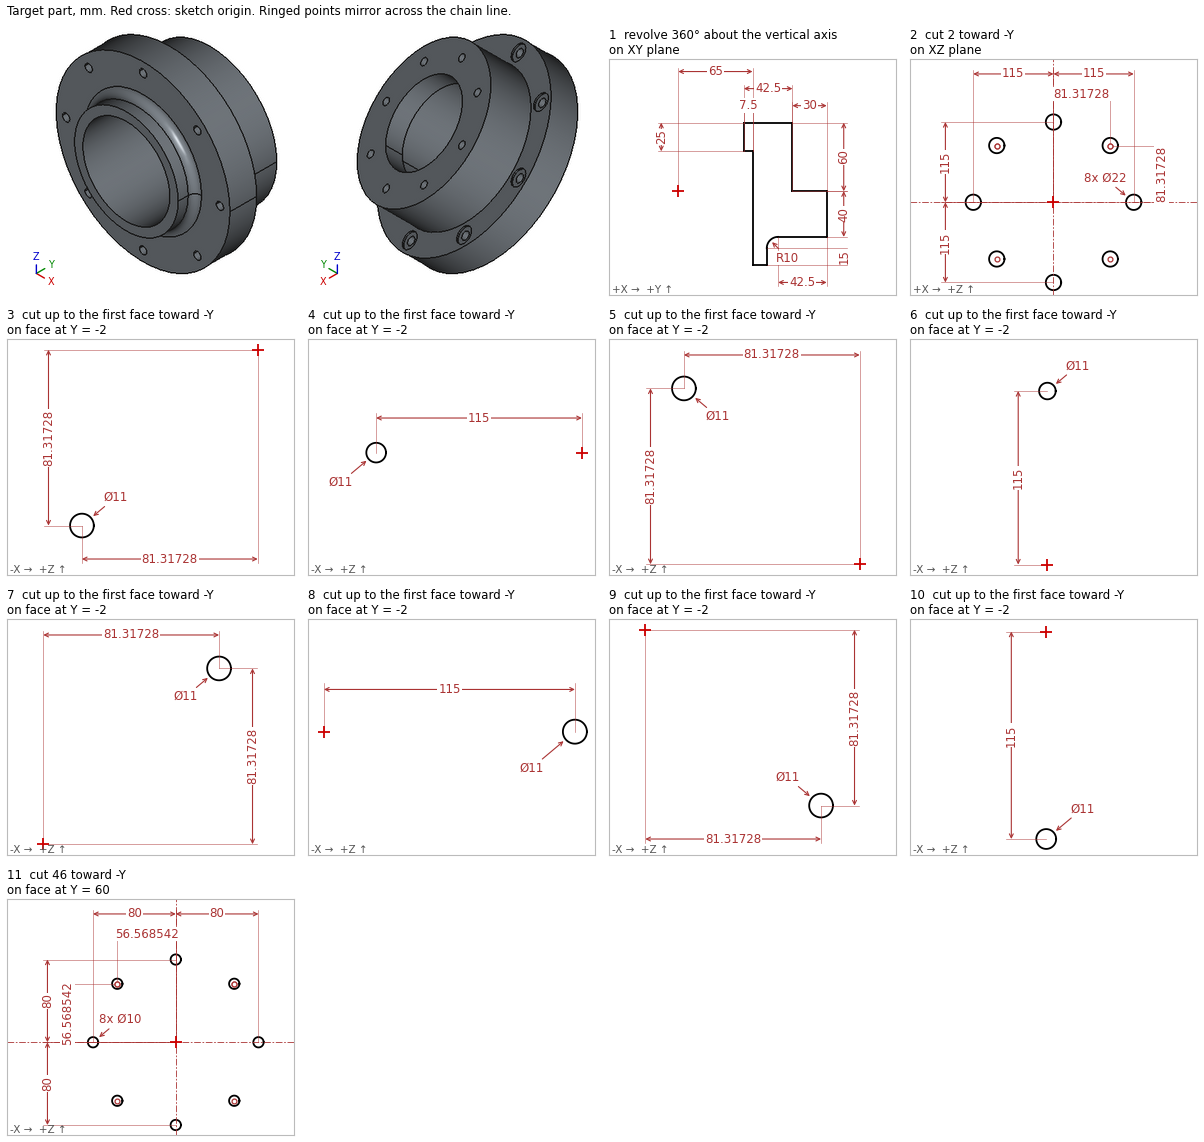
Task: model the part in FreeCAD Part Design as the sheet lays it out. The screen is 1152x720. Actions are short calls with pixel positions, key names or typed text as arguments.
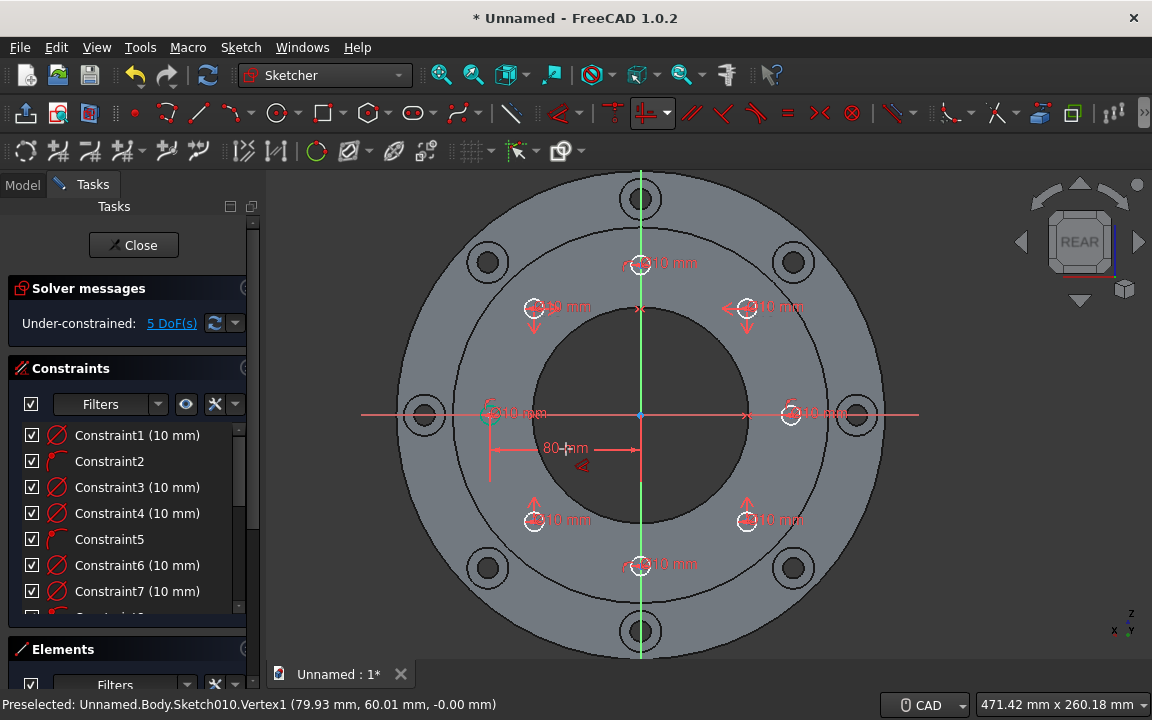
click(641, 265)
click(675, 340)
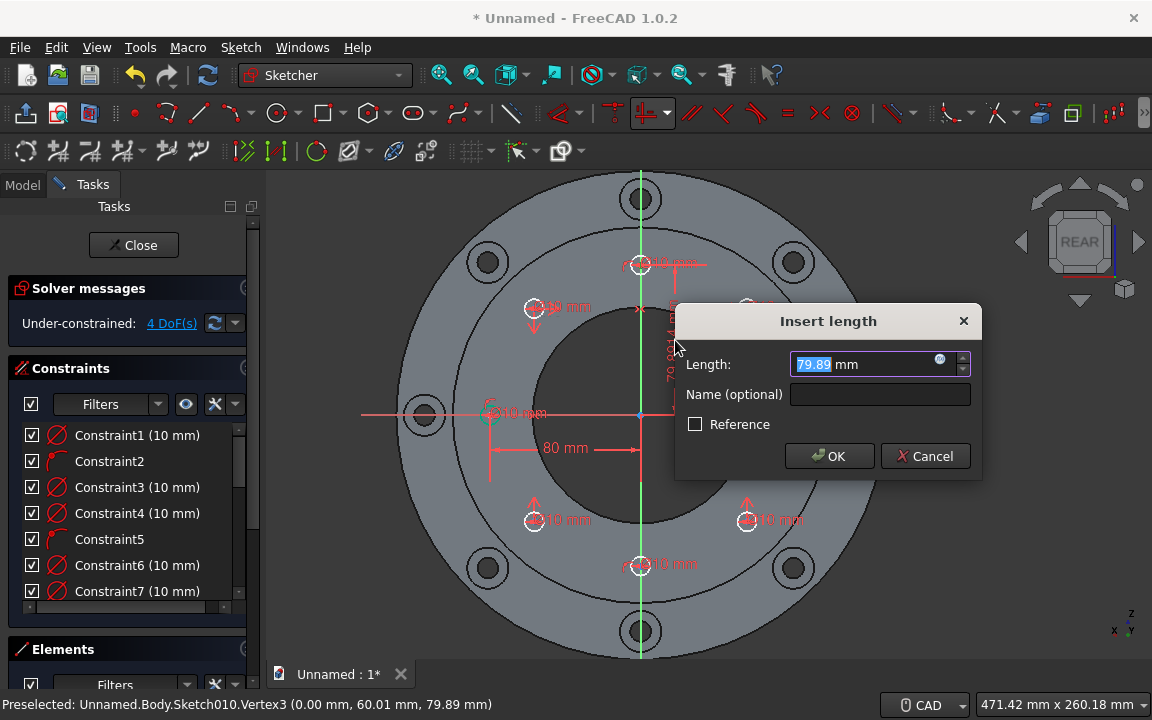
text(80)
key(Return)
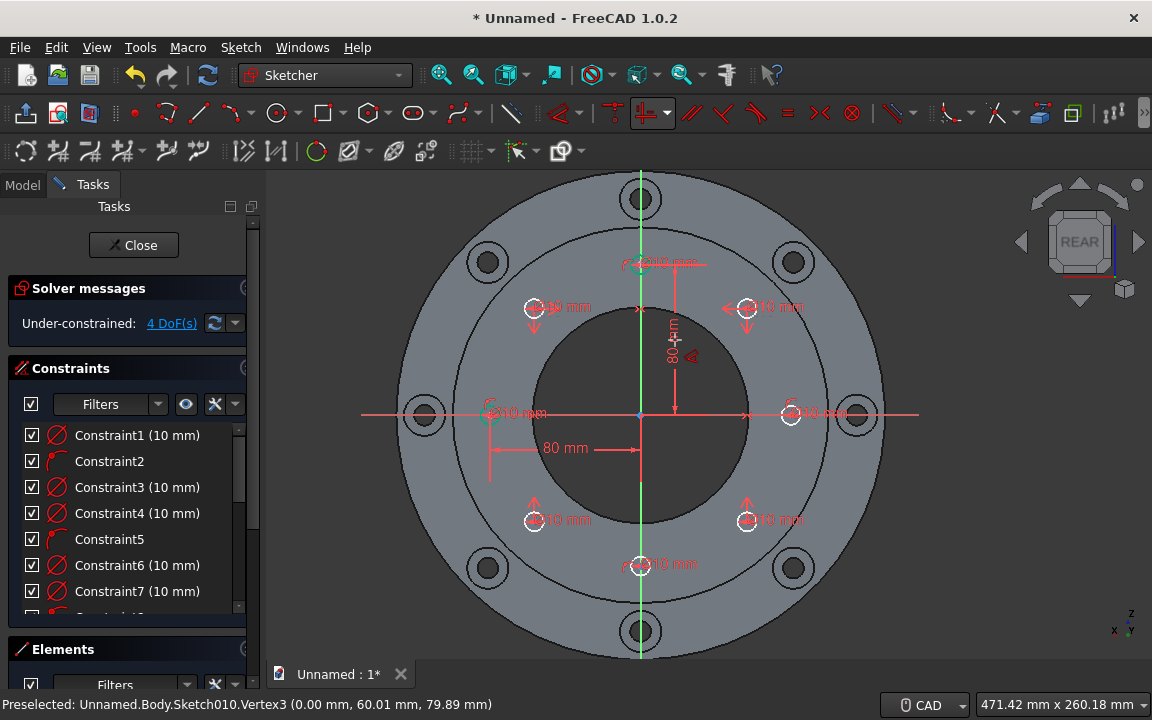
click(791, 415)
click(716, 449)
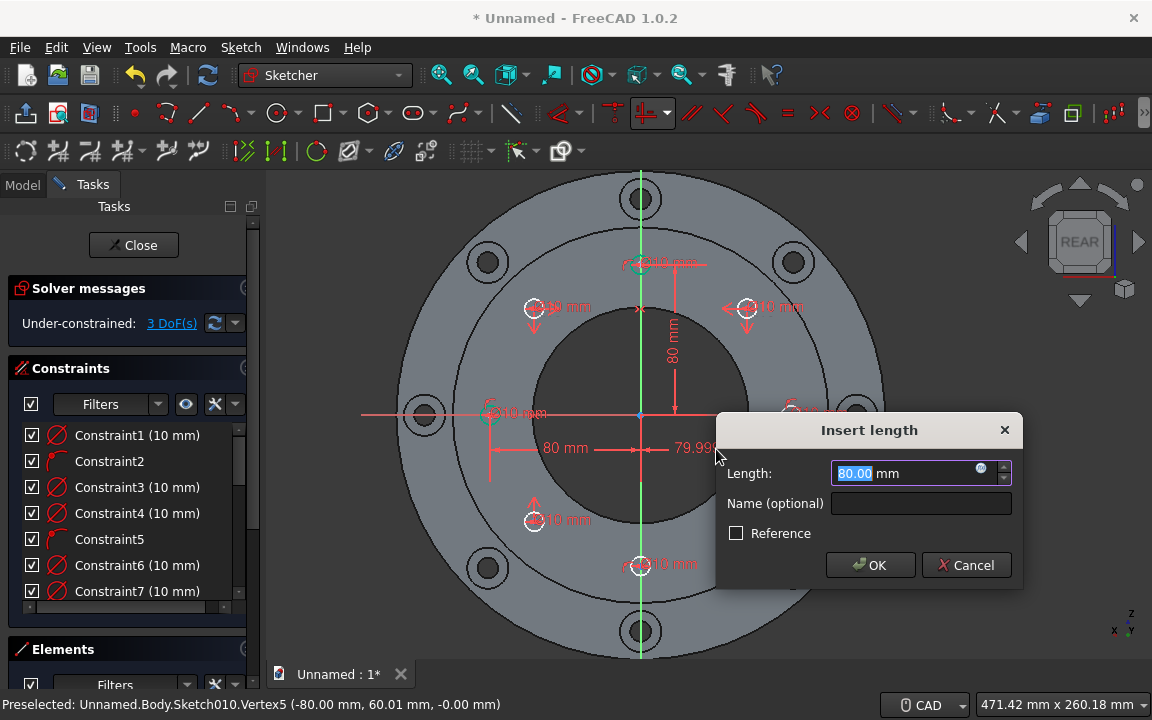
text(80)
key(Return)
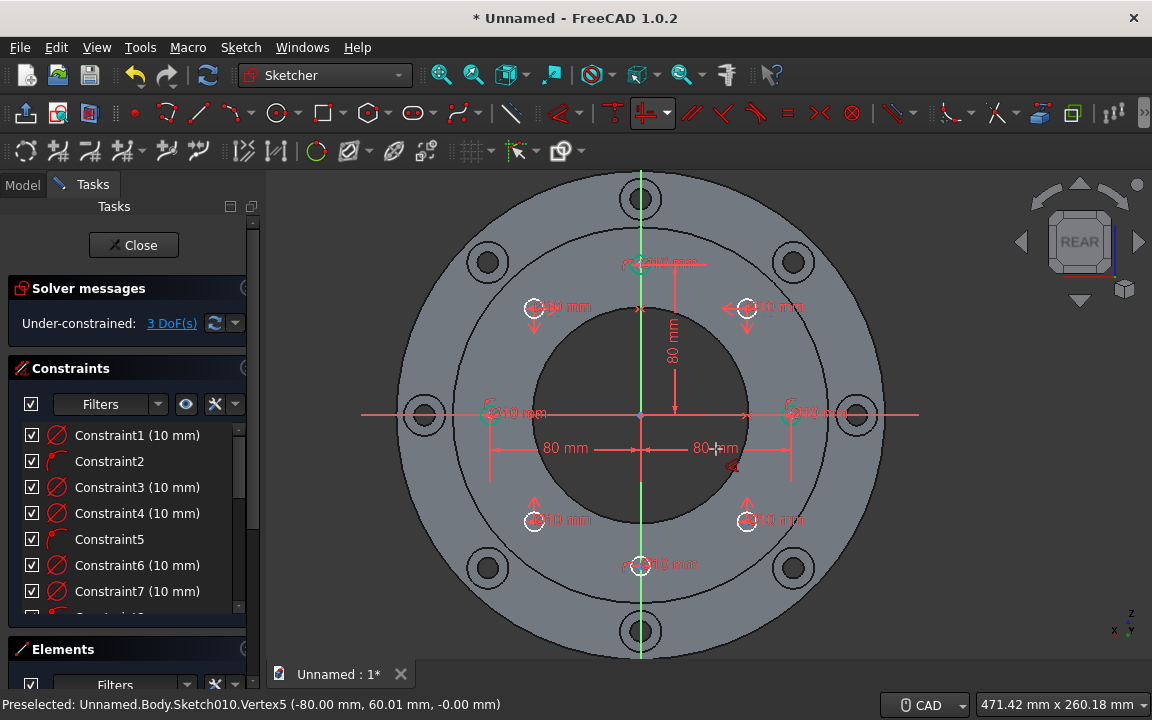
click(641, 566)
click(675, 491)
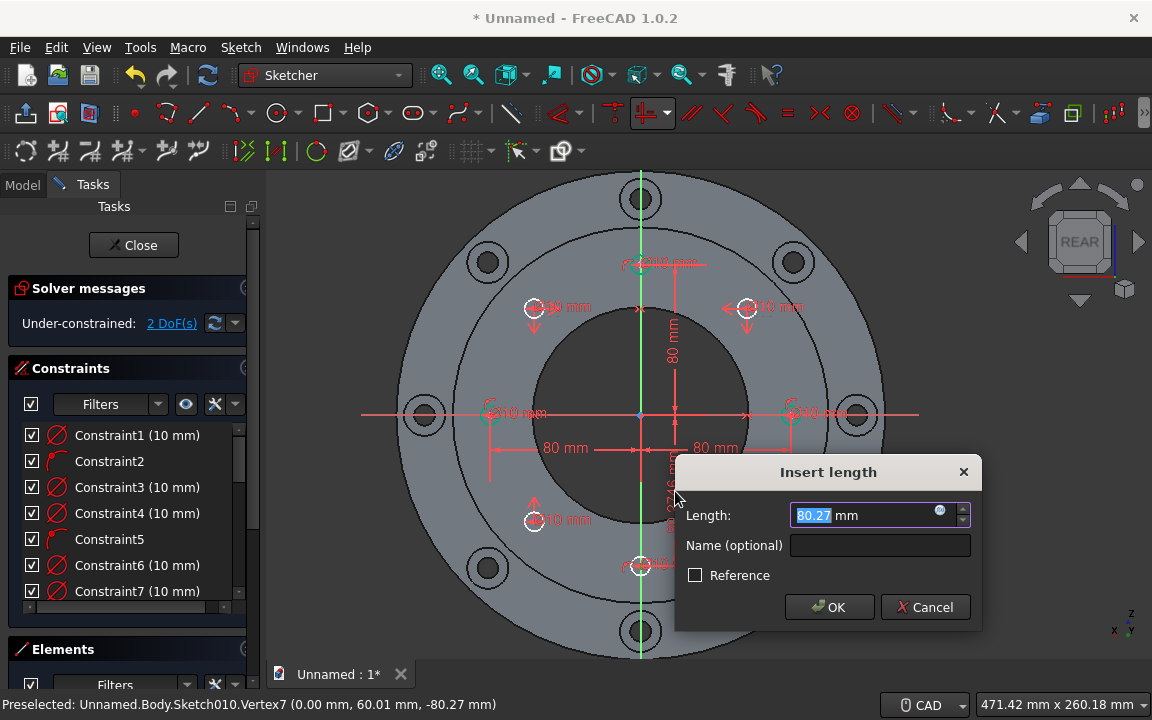
text(80)
key(Return)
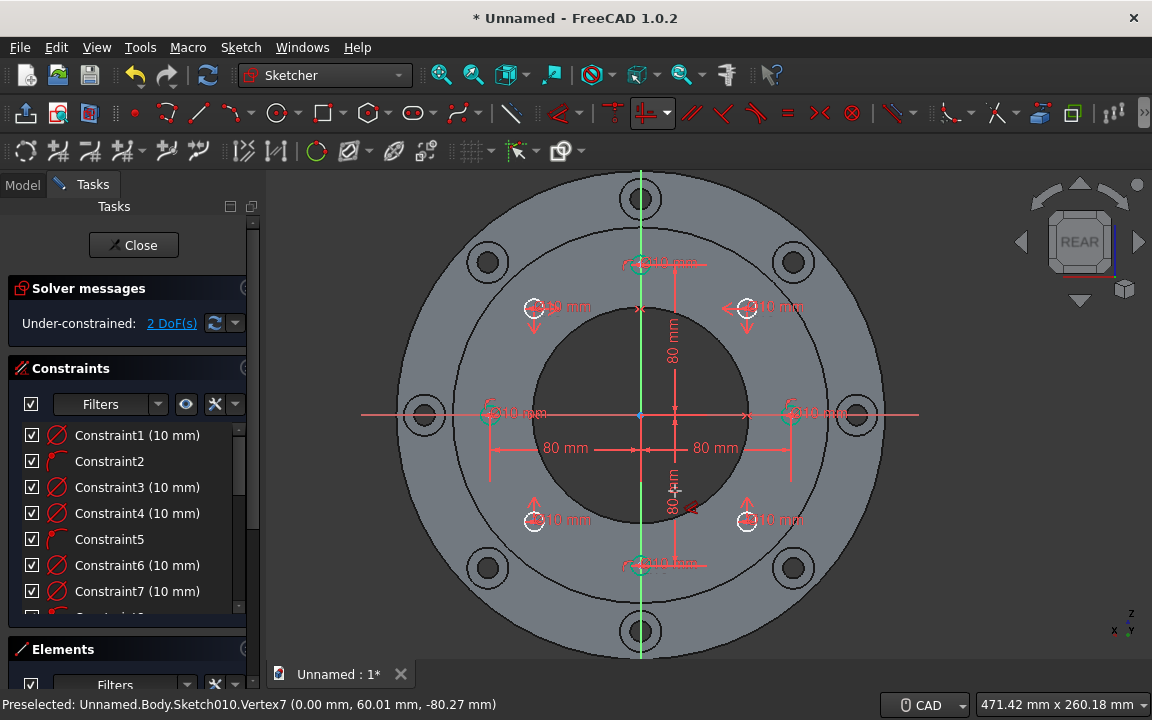
click(534, 309)
click(587, 275)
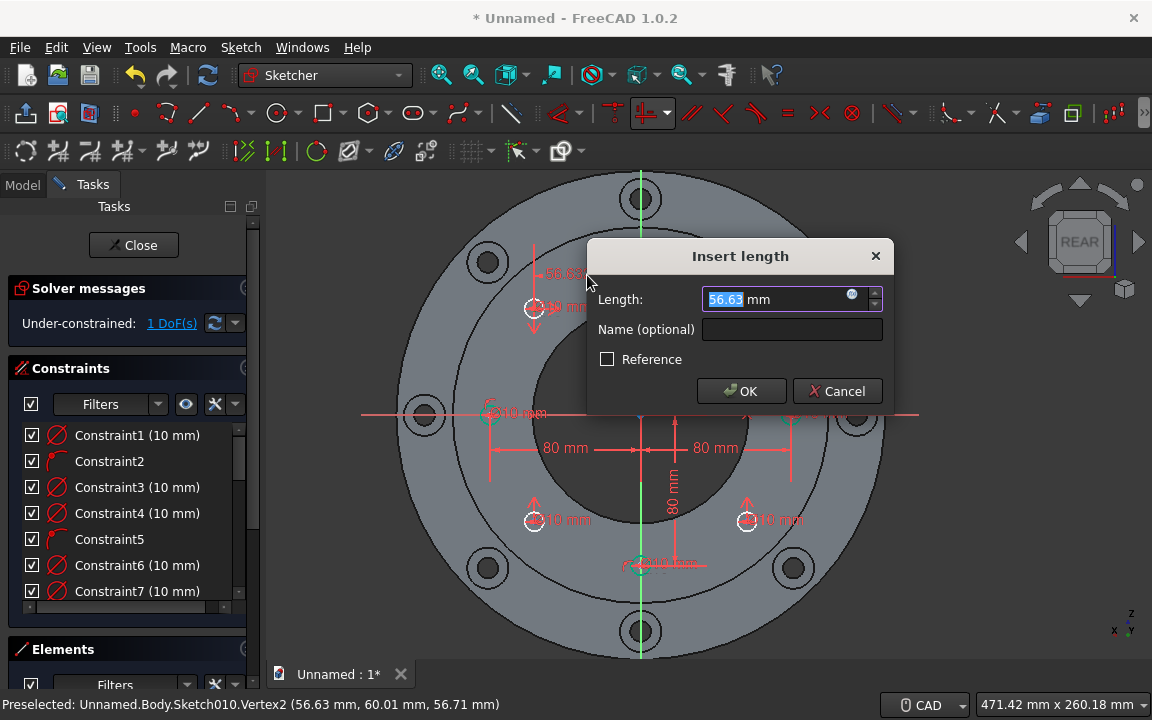
text(56.568542)
key(Return)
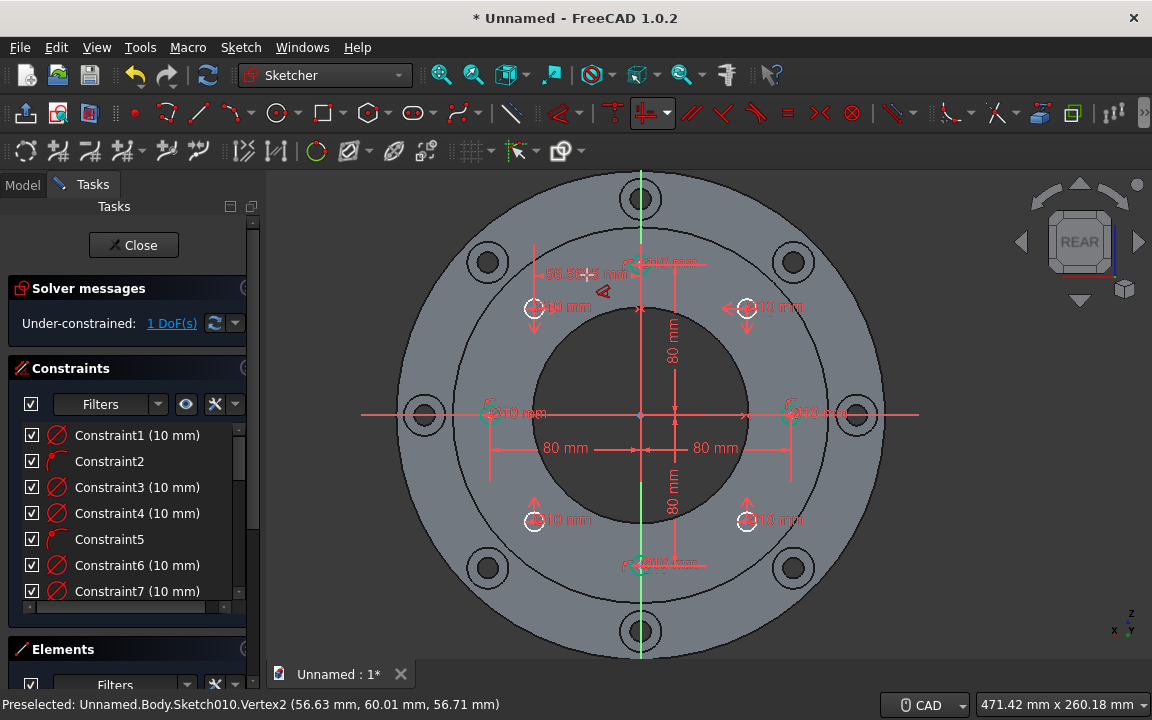
click(534, 309)
click(500, 362)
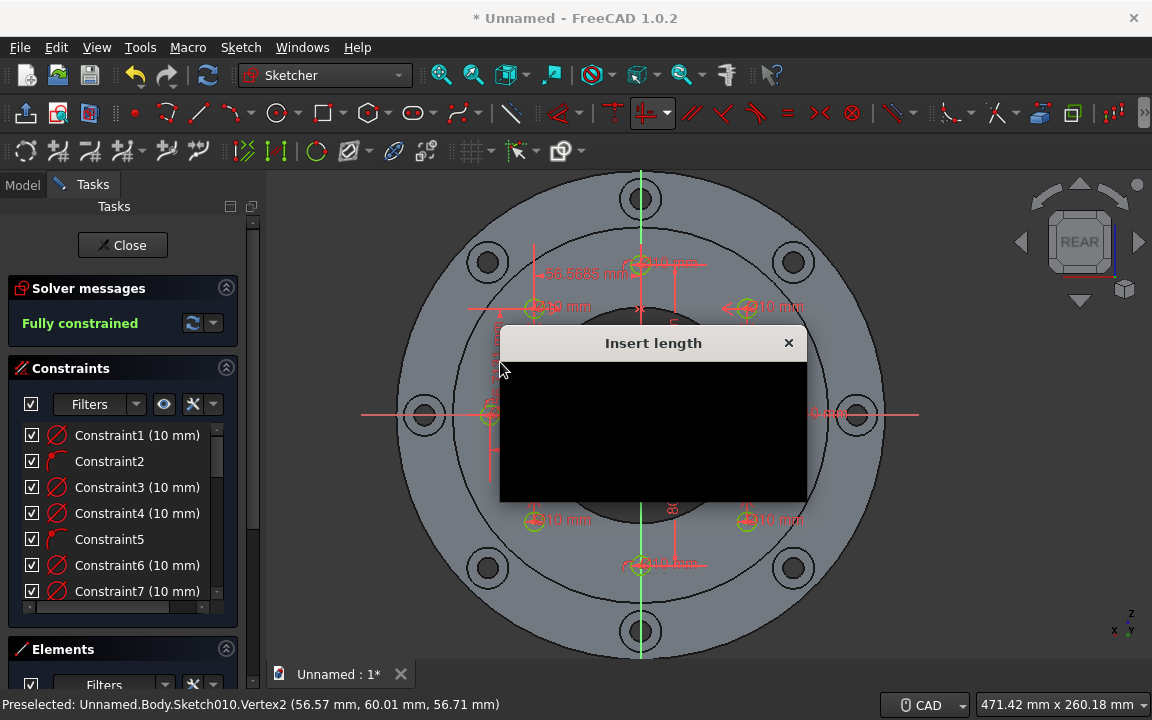
text(56.568542)
key(Return)
key(Escape)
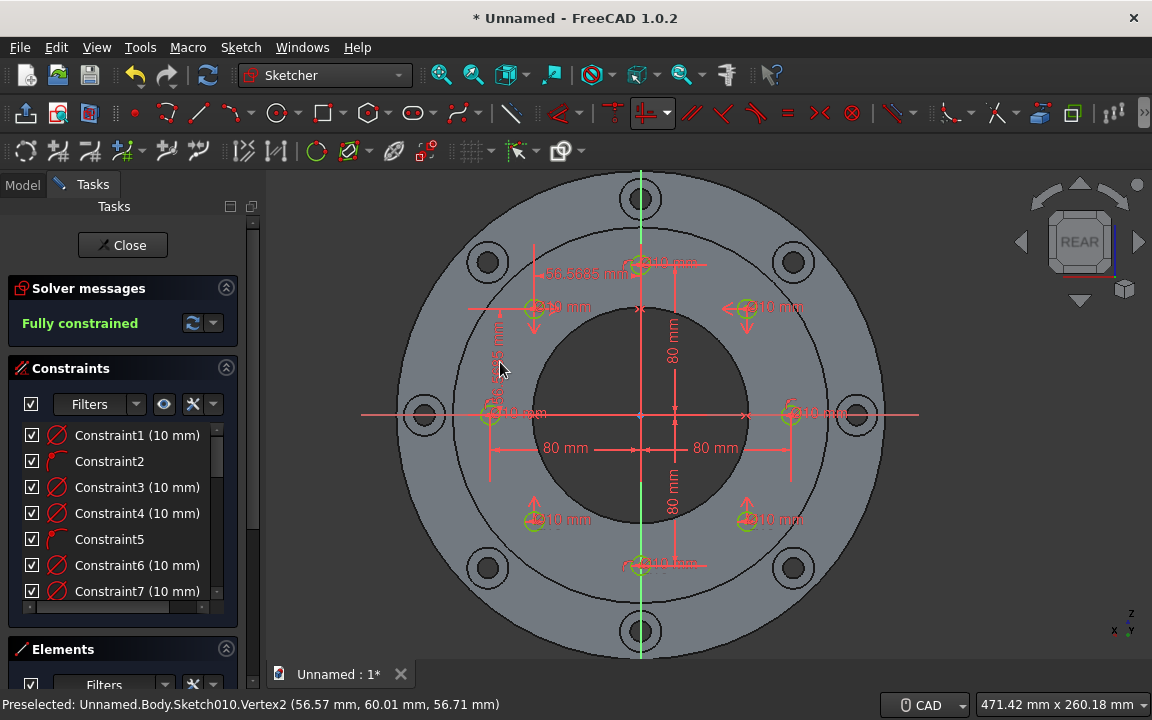
click(123, 245)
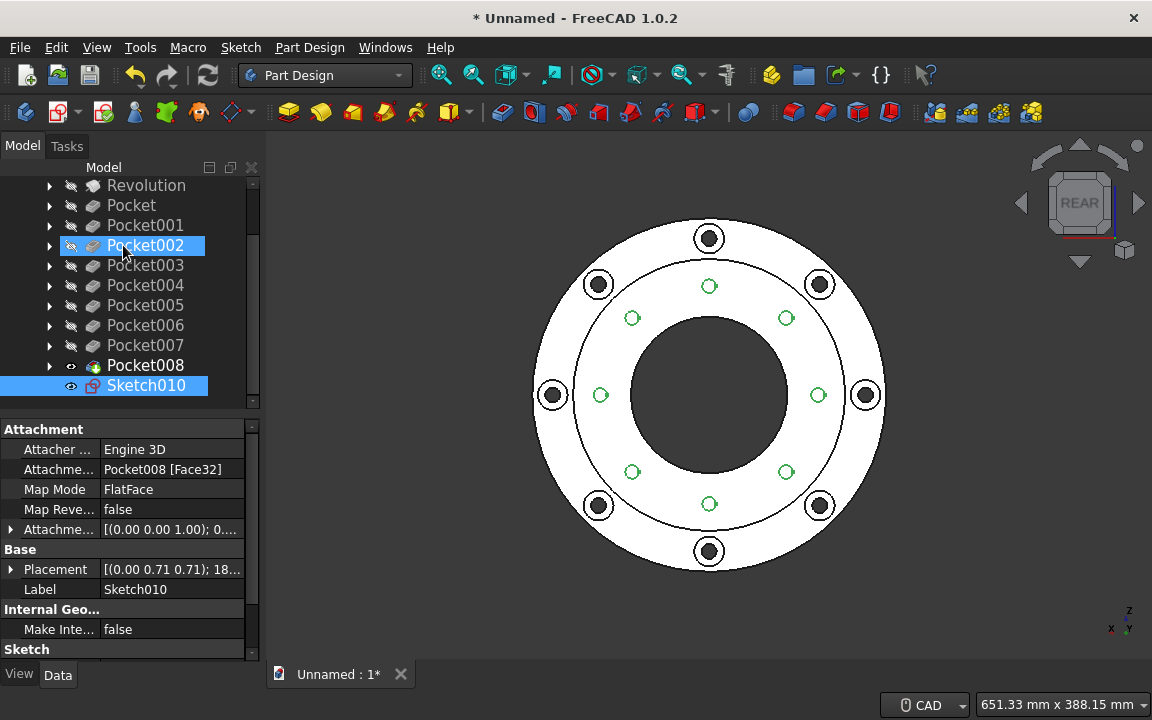
click(504, 112)